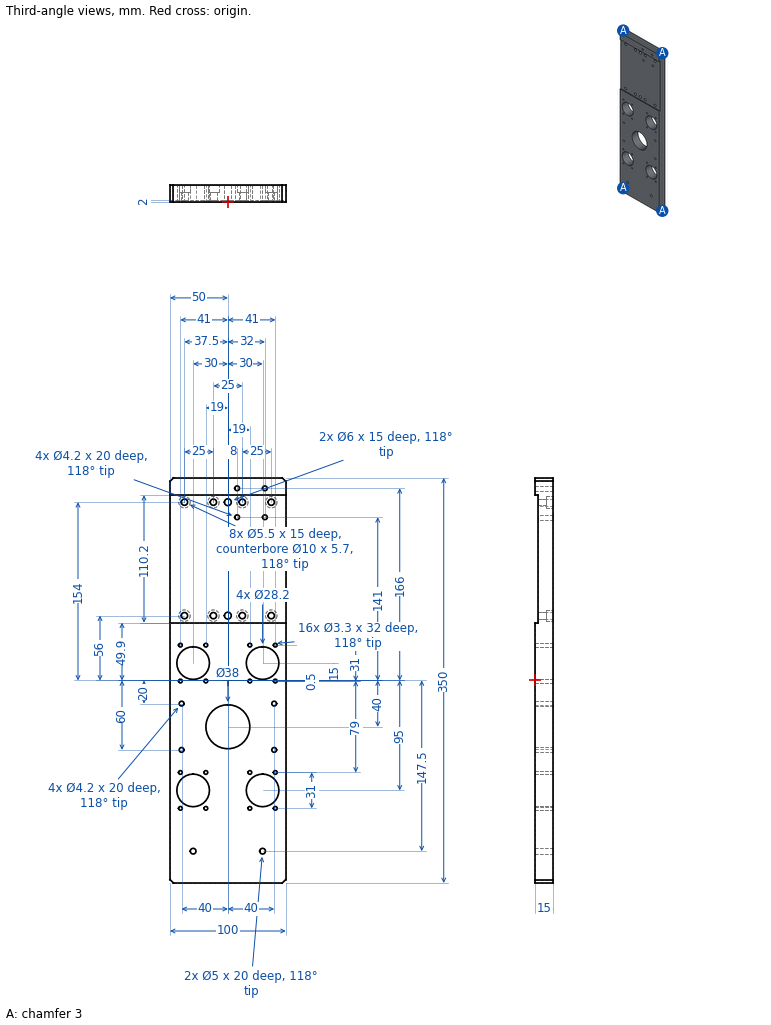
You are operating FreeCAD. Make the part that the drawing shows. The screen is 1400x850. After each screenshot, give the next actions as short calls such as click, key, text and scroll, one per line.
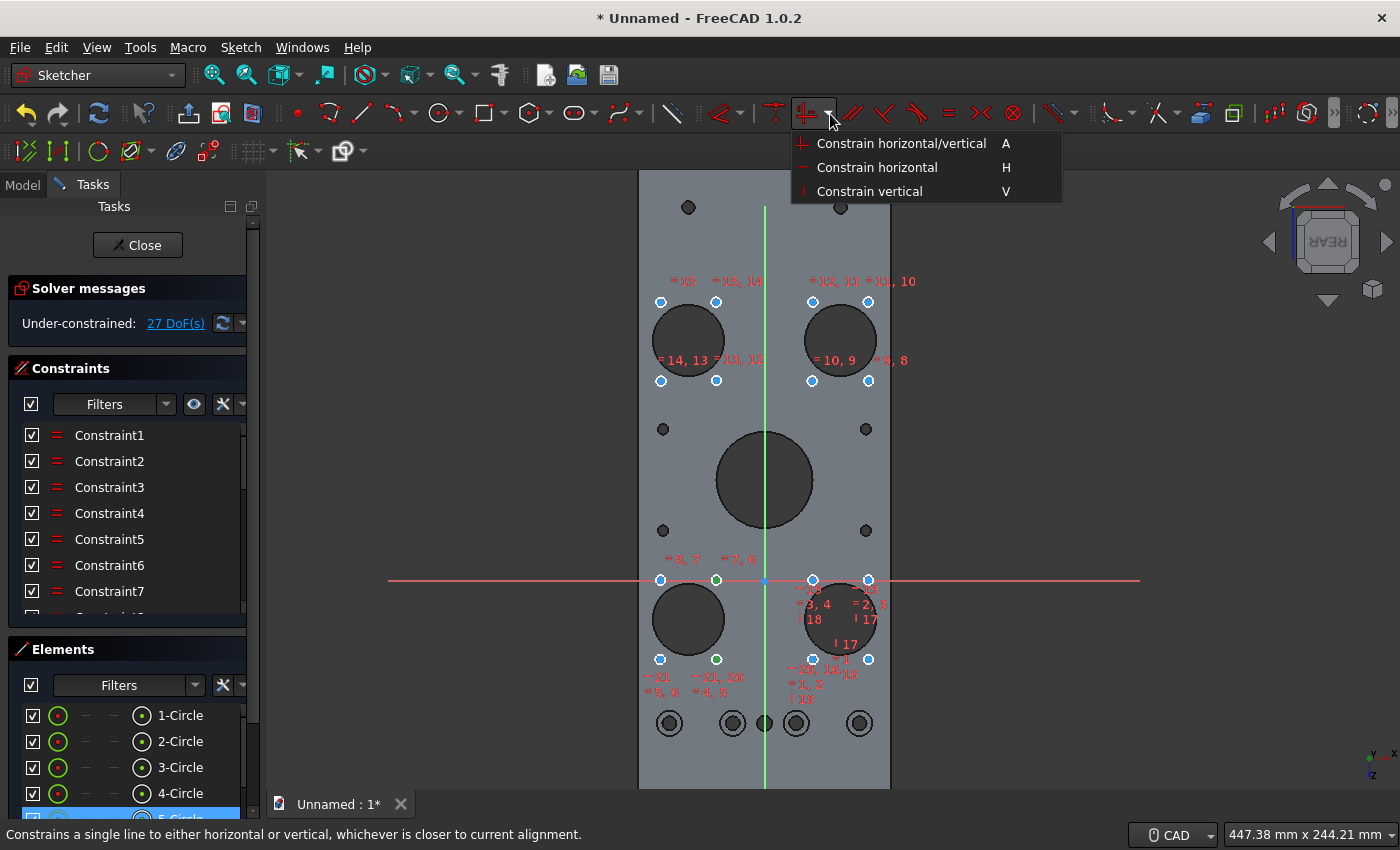
click(927, 191)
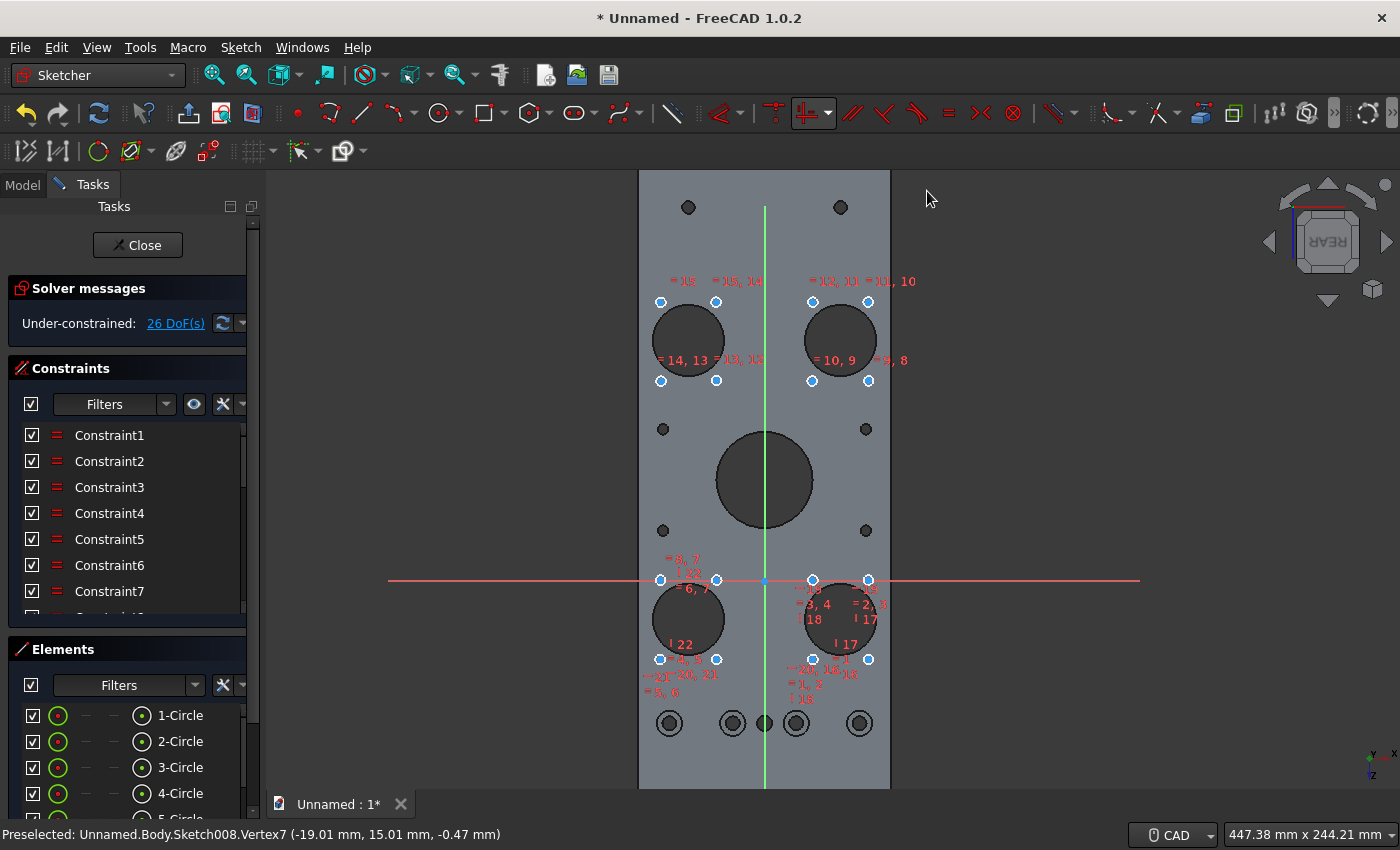
click(813, 580)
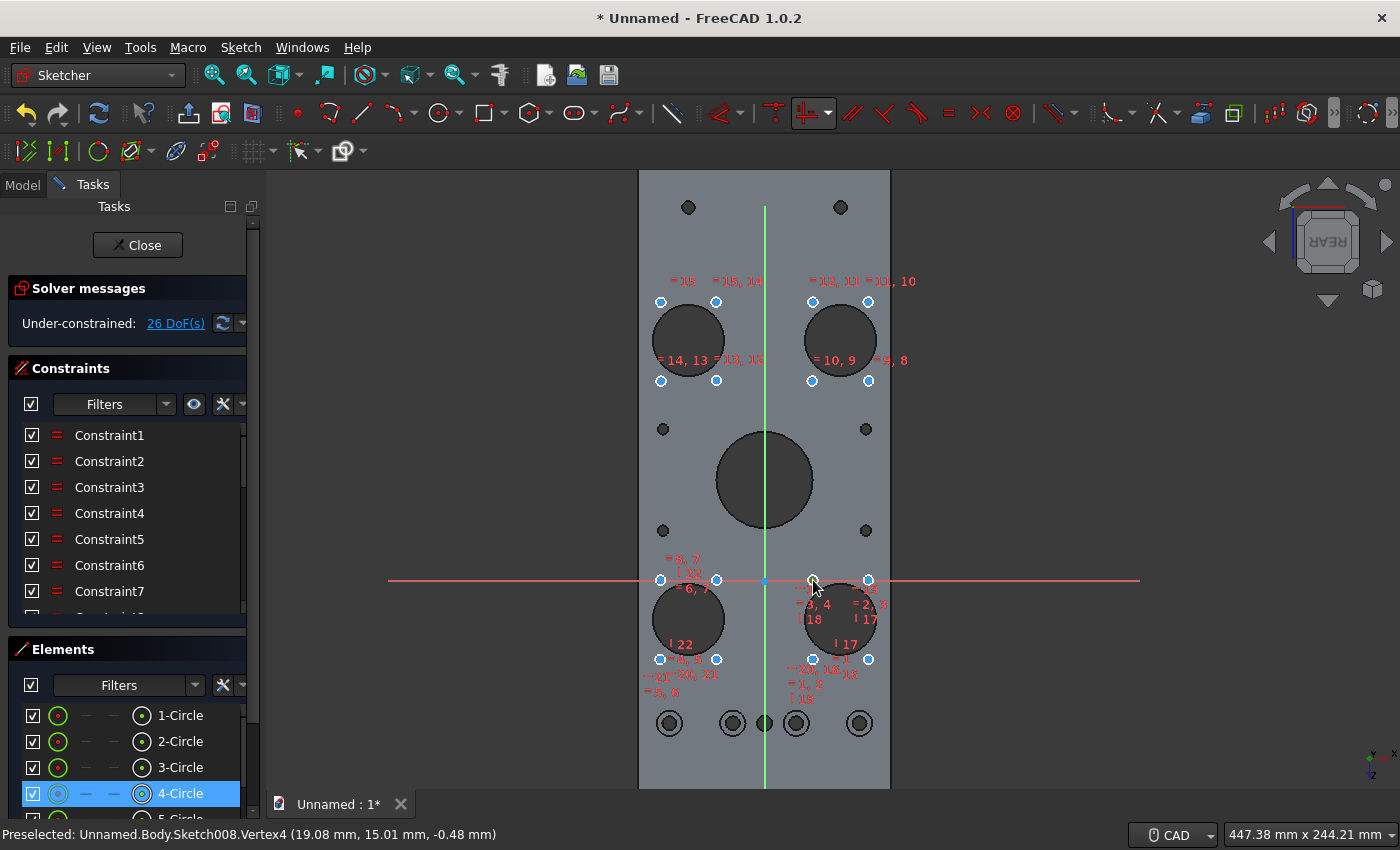
click(717, 580)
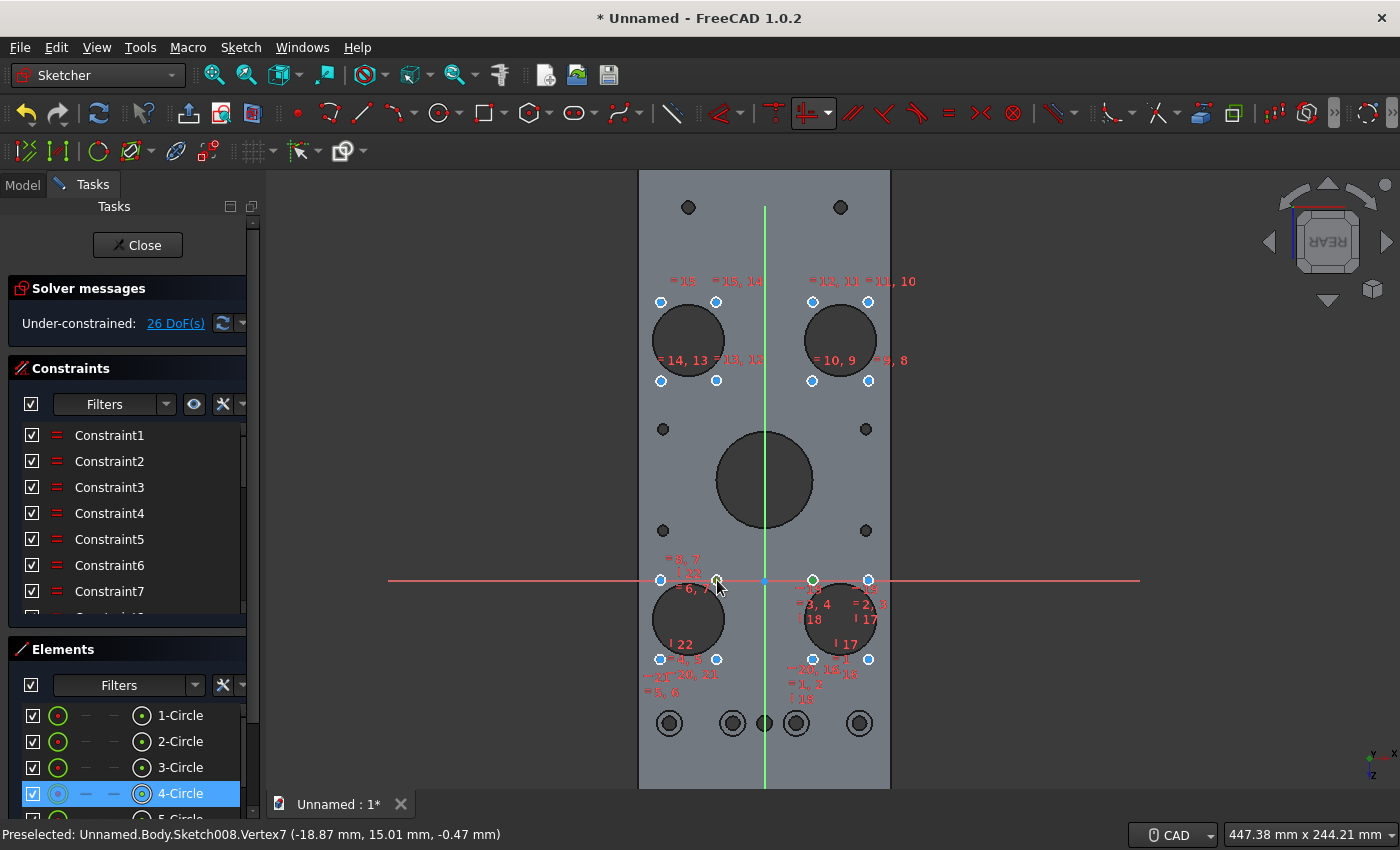
key(h)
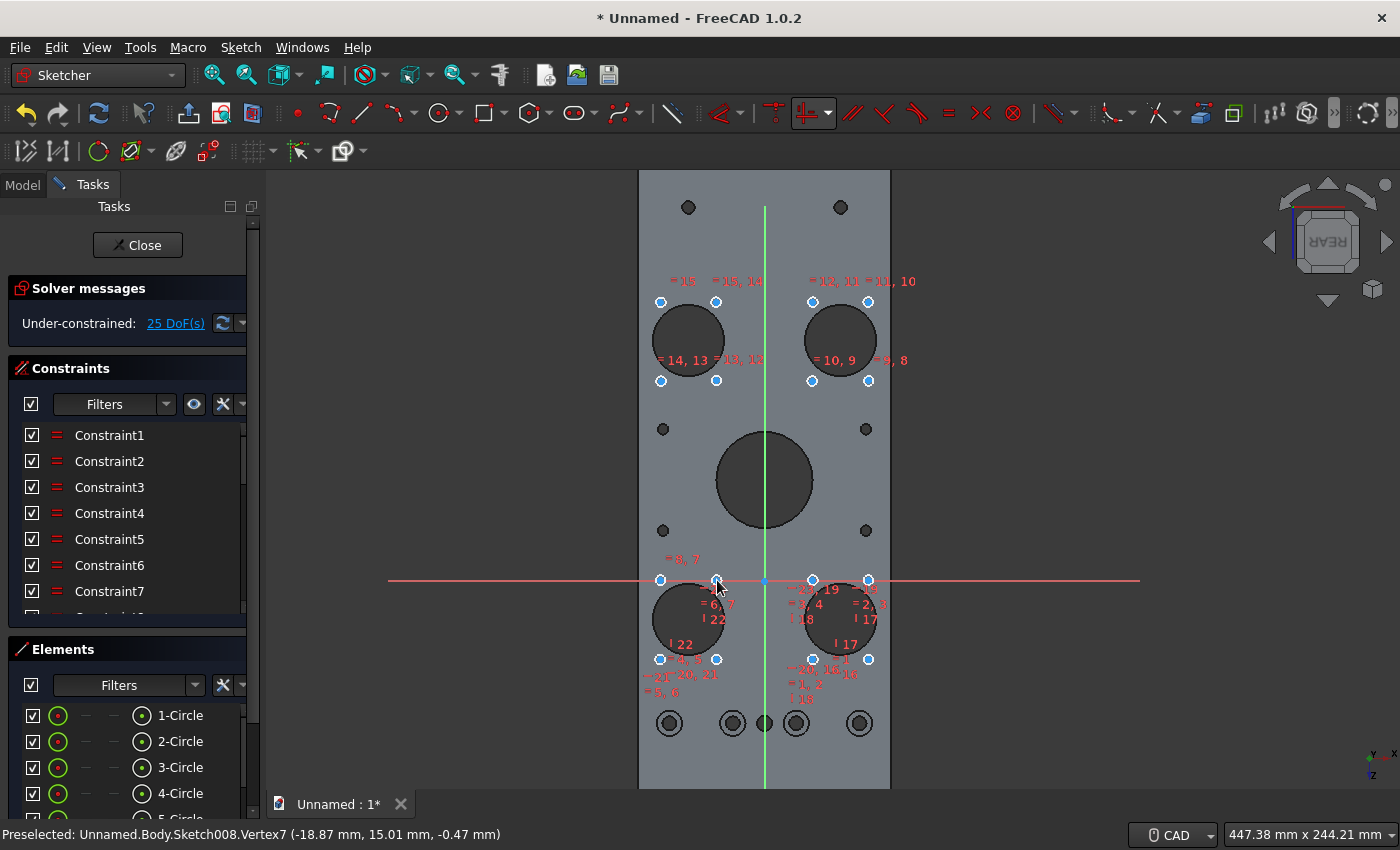
click(660, 660)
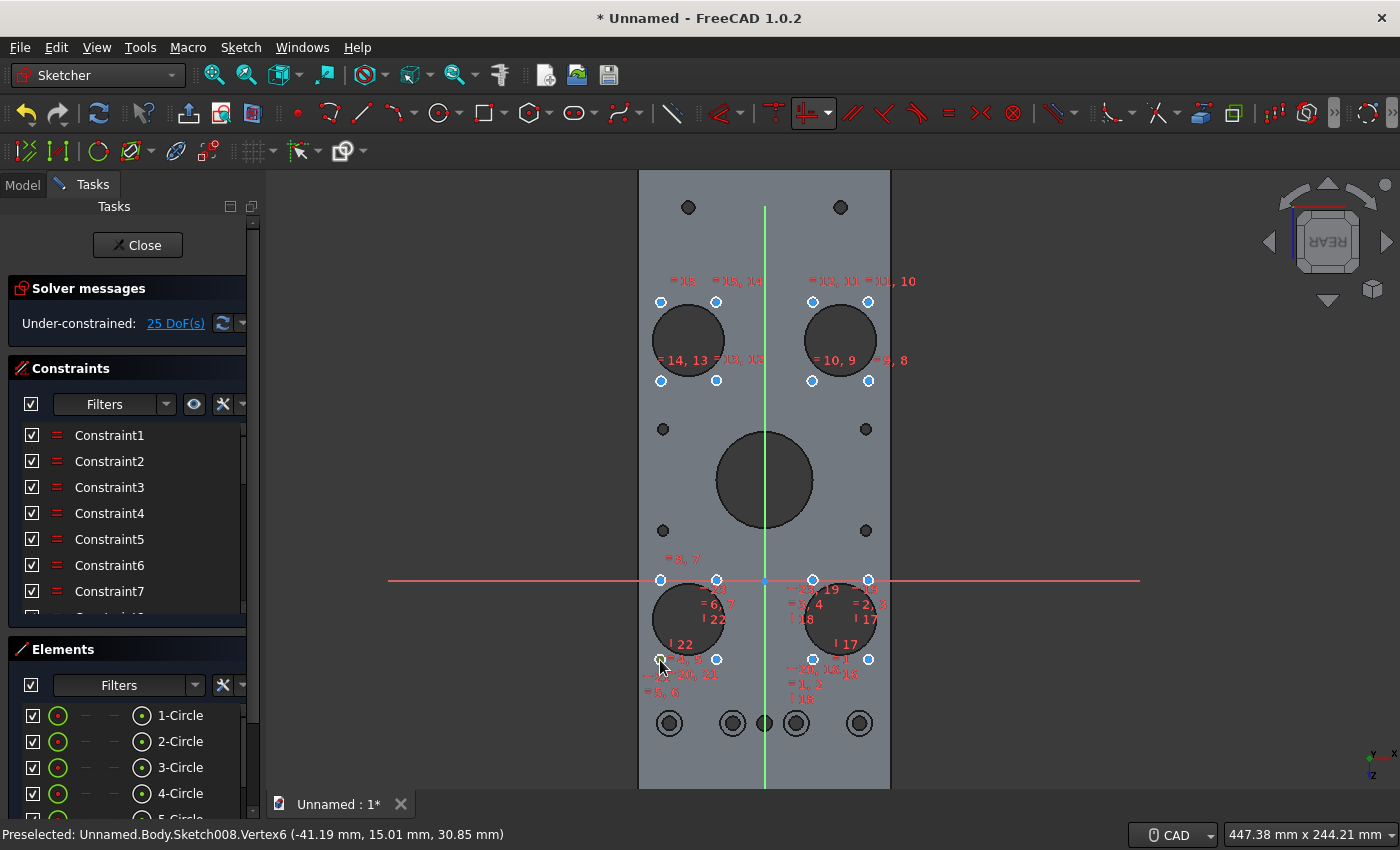
click(661, 580)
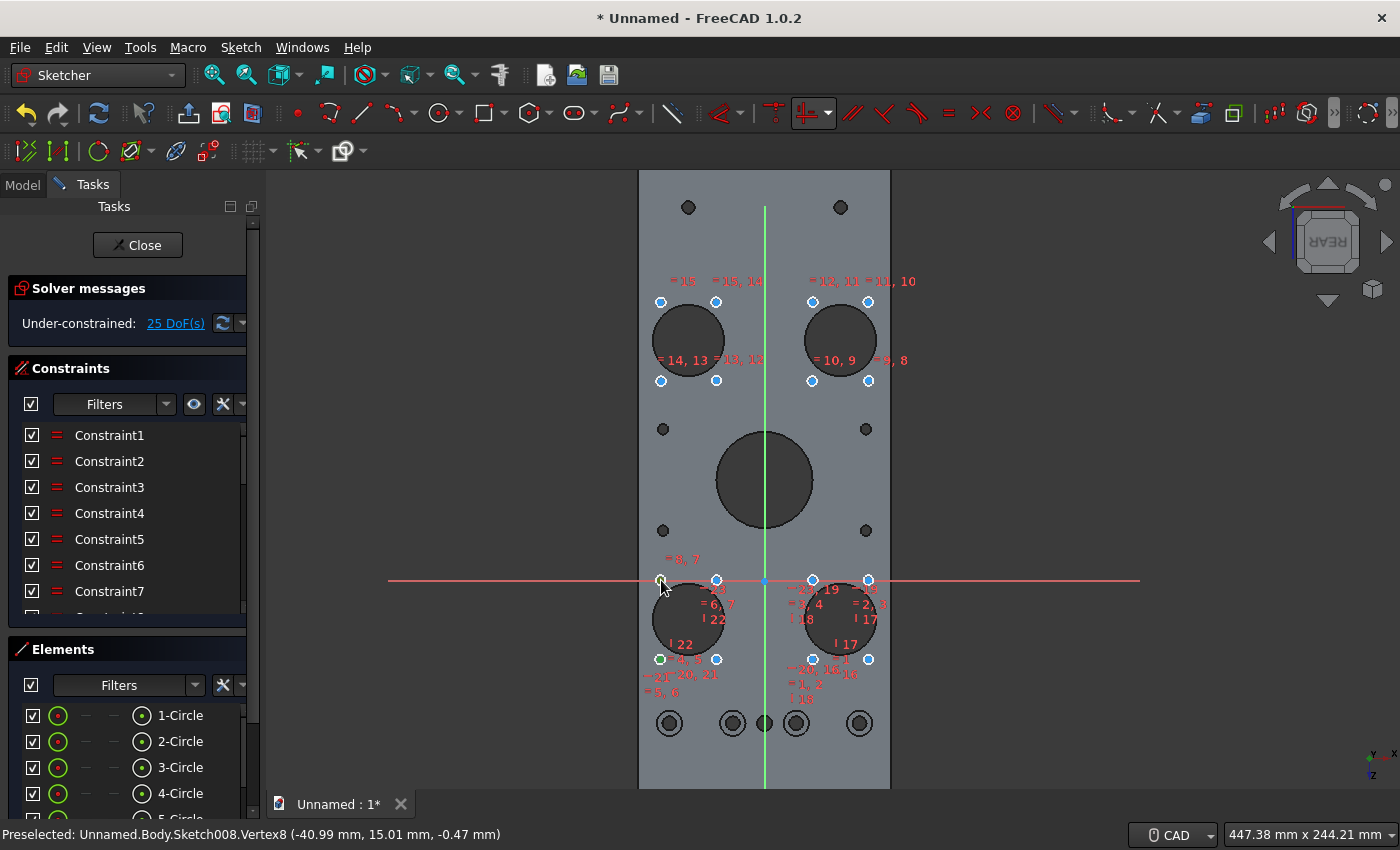
key(v)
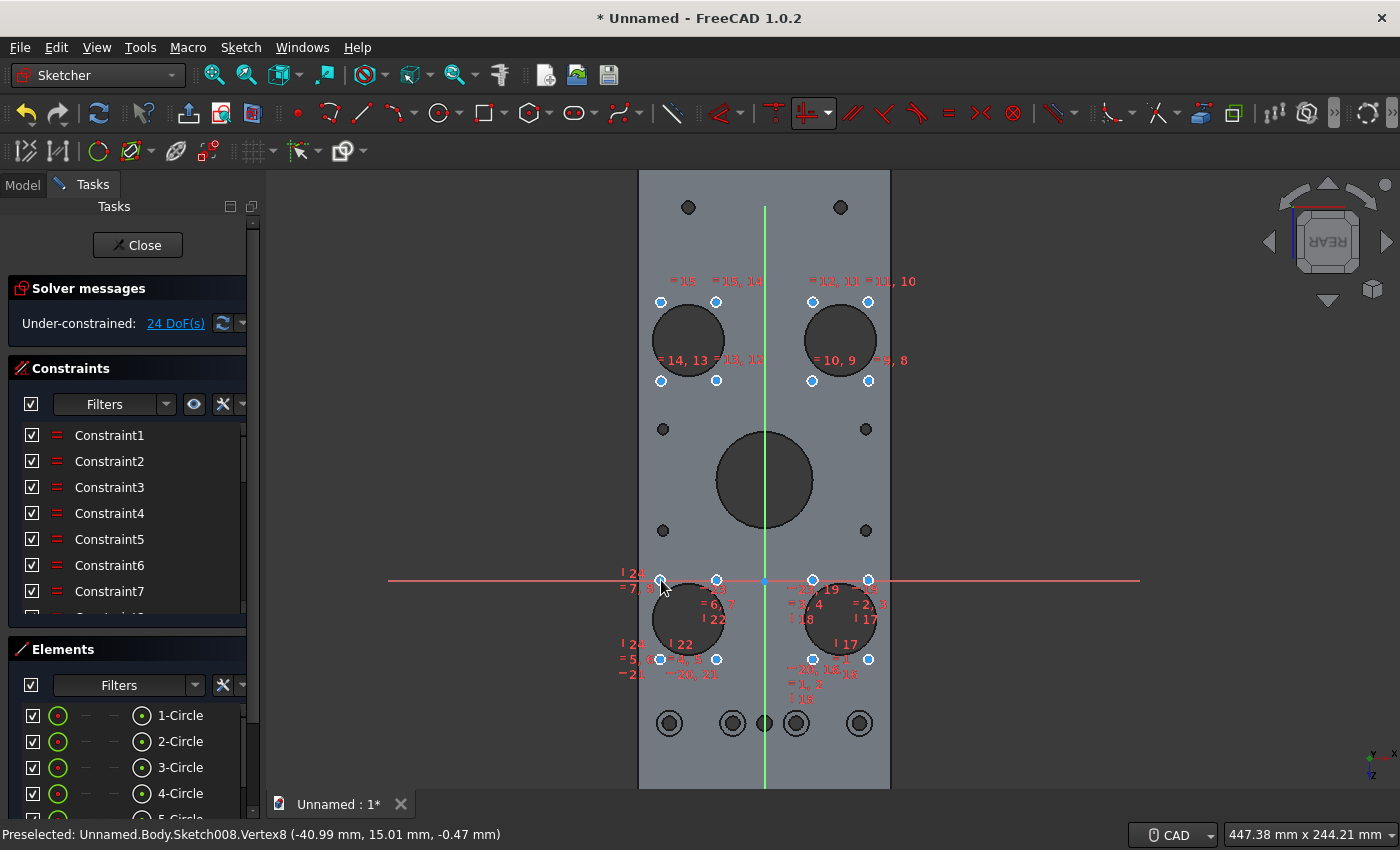
click(717, 580)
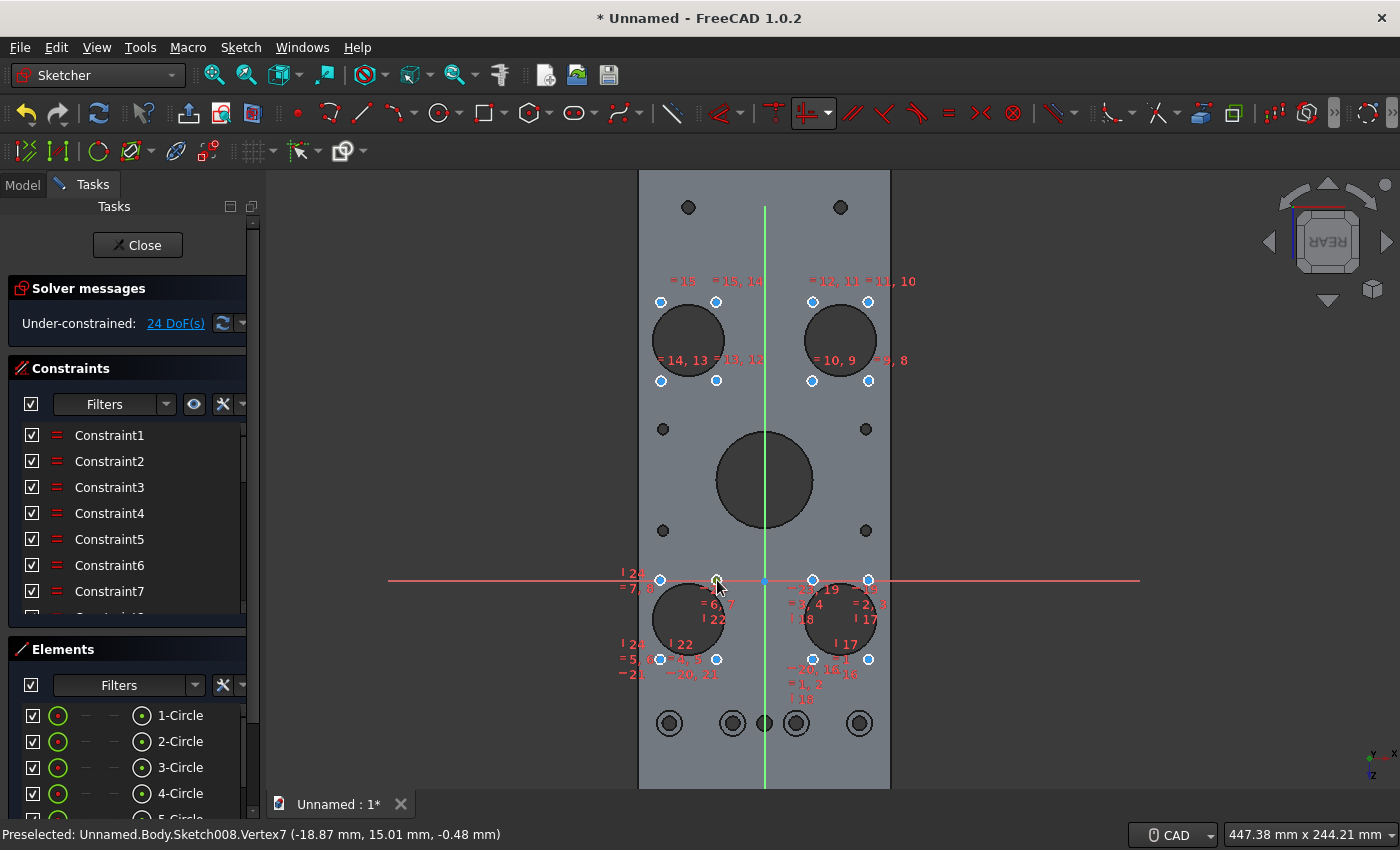
click(660, 580)